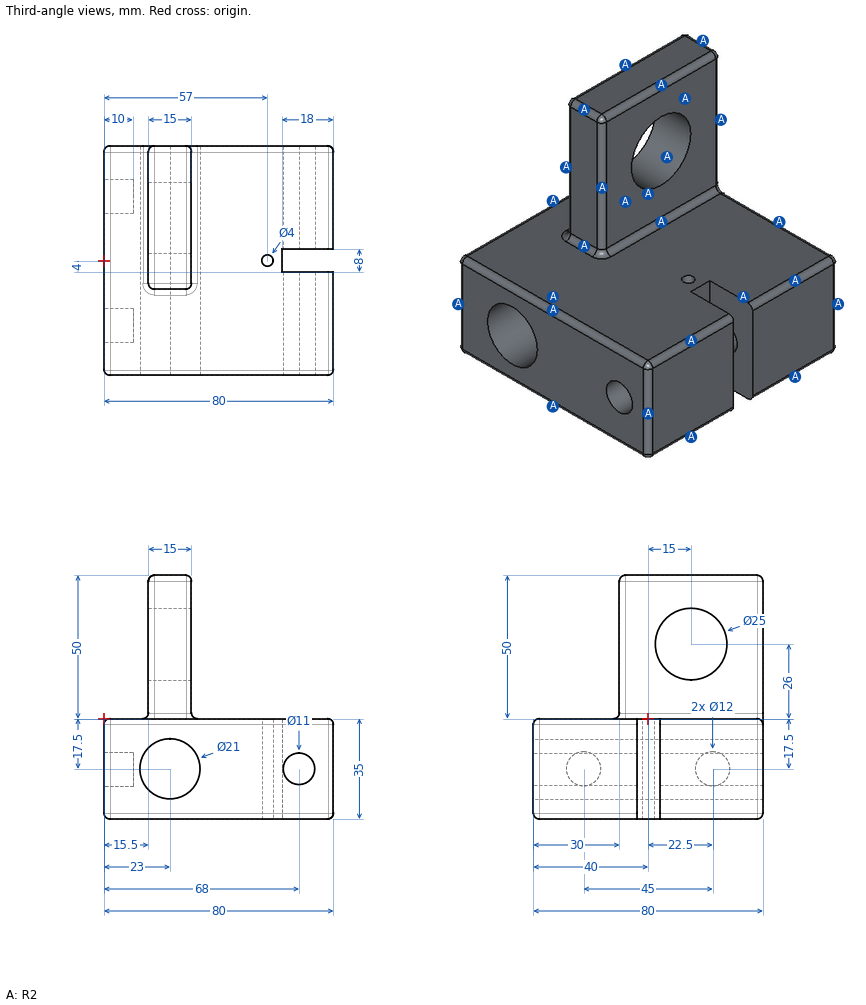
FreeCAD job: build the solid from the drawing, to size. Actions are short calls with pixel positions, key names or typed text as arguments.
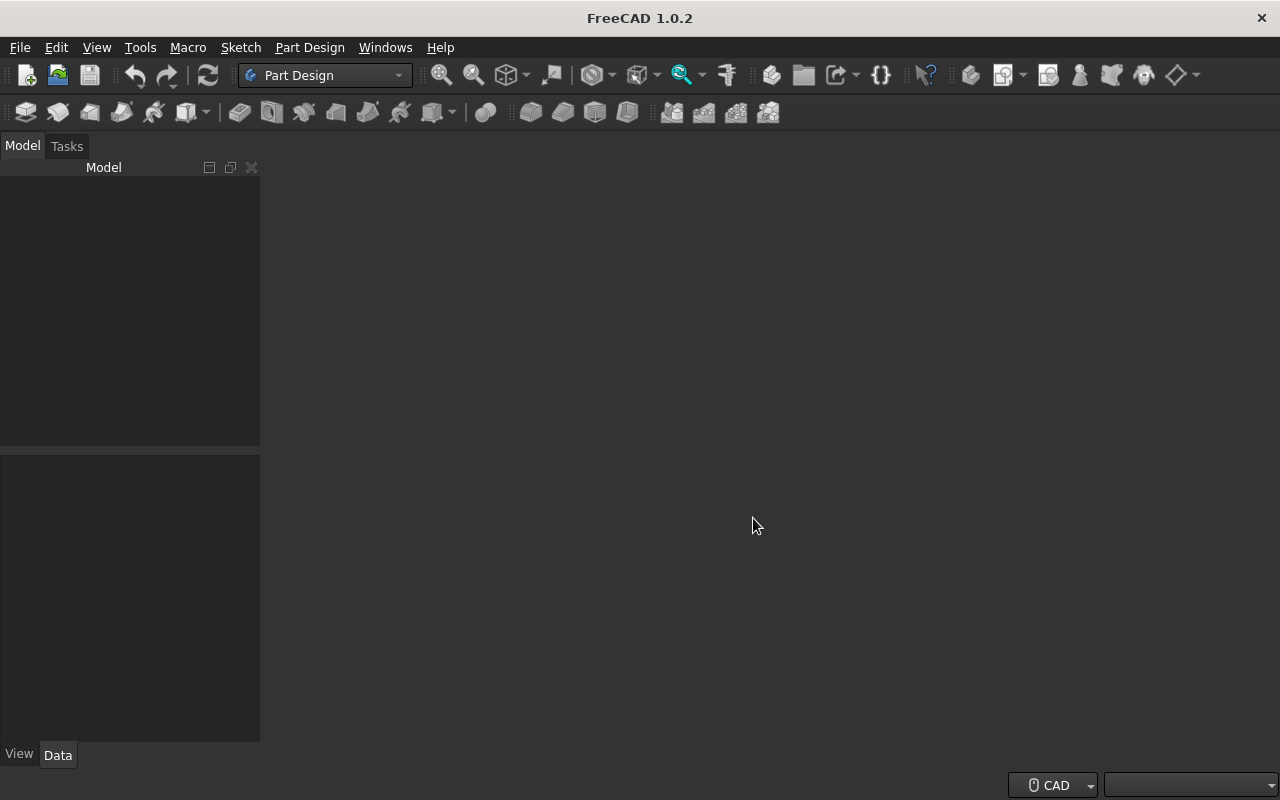
click(26, 76)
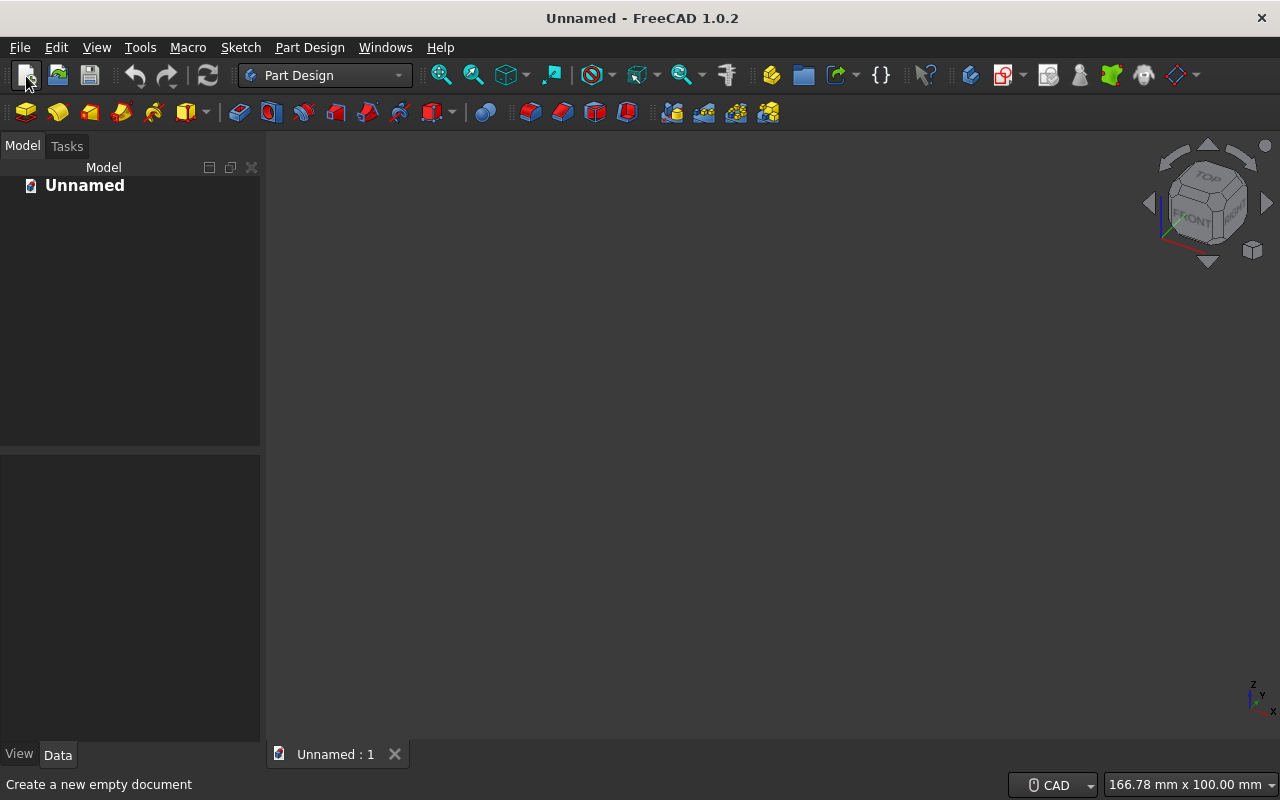
click(1004, 76)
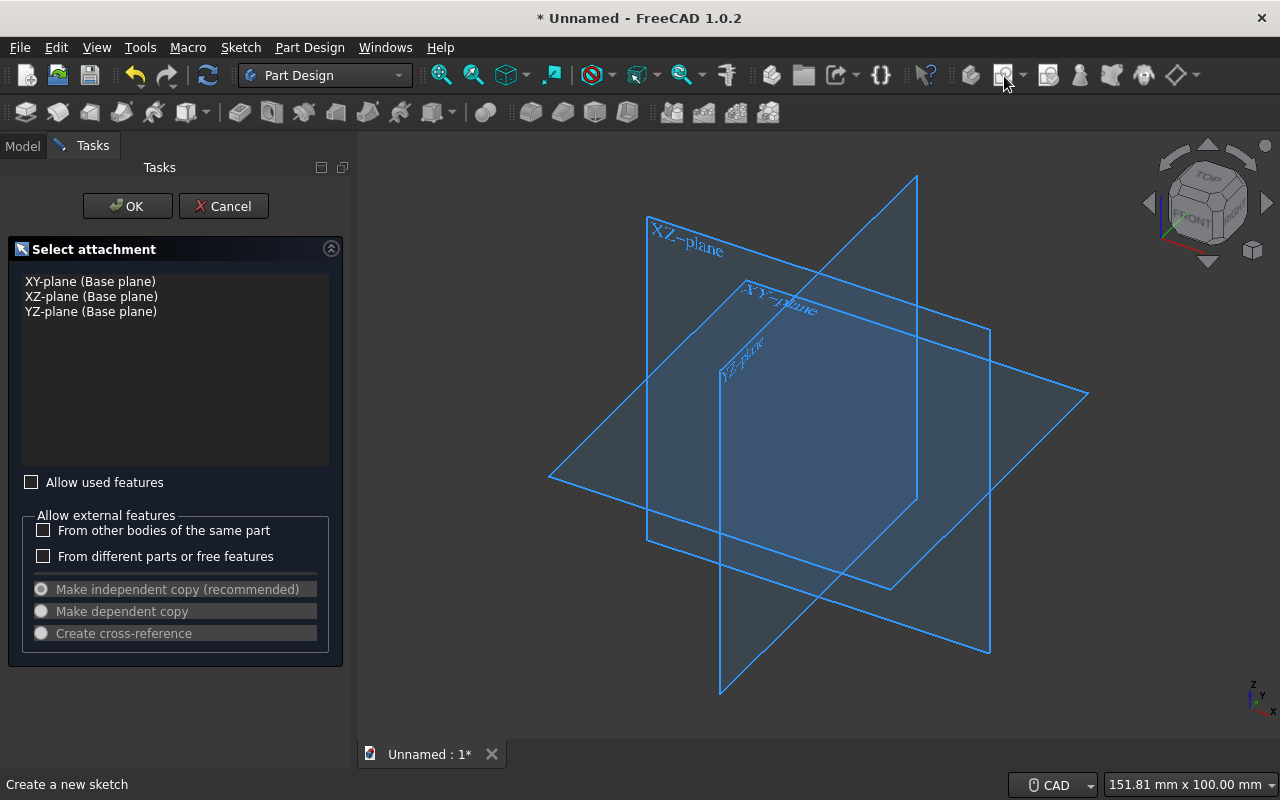
click(82, 296)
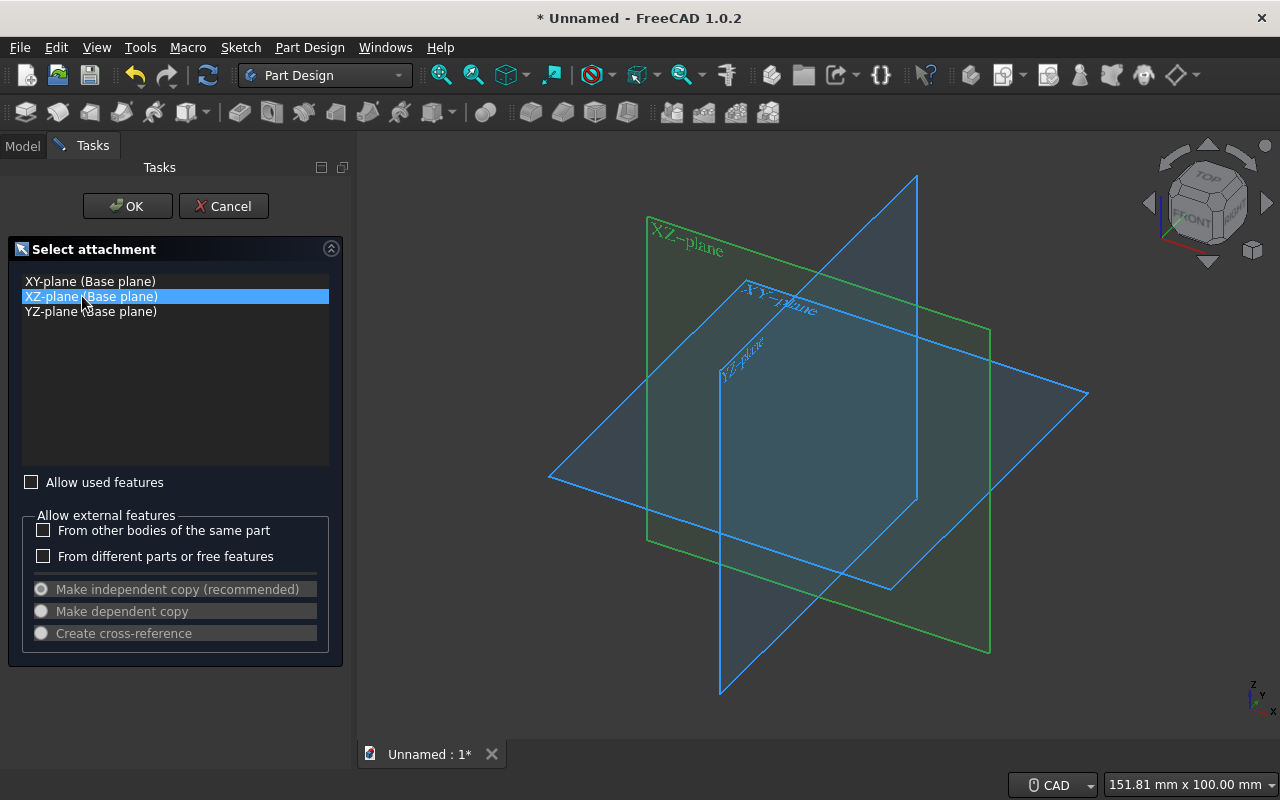
click(128, 206)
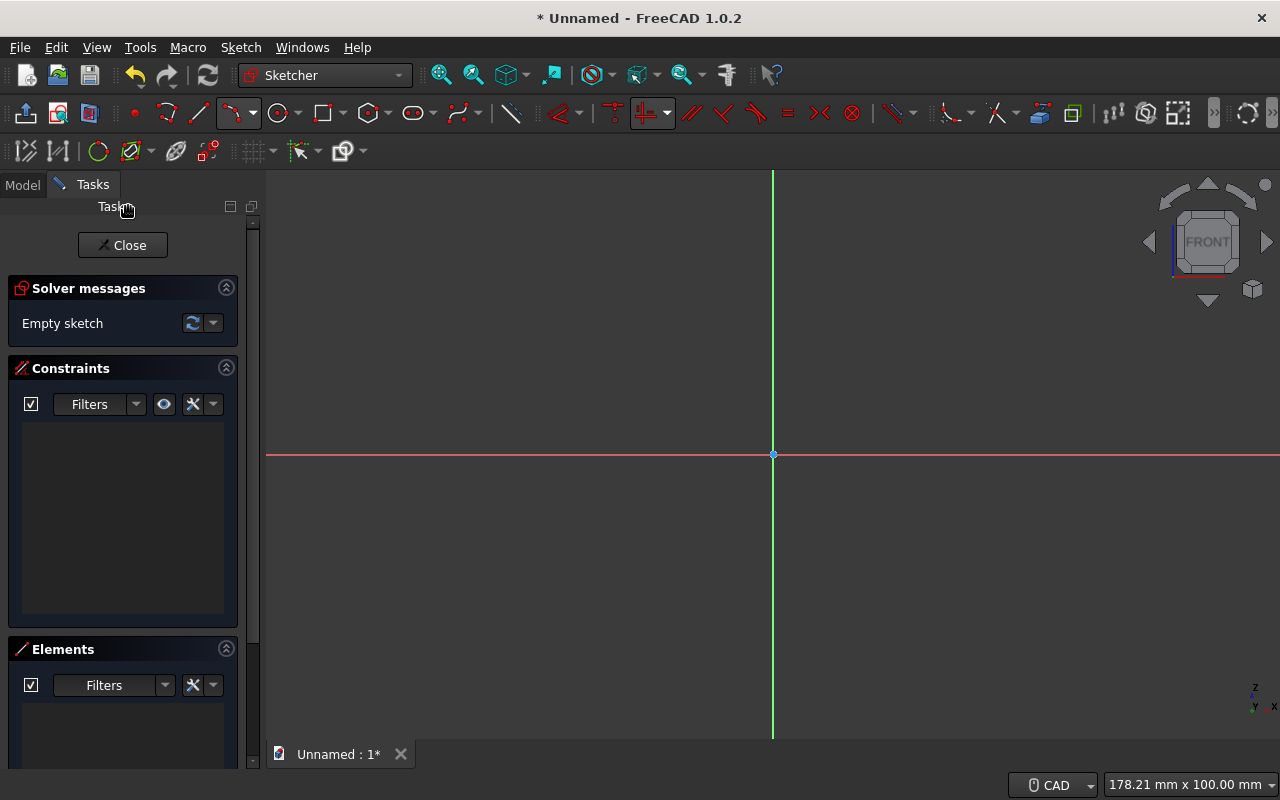
scroll(294, 647, down, 1)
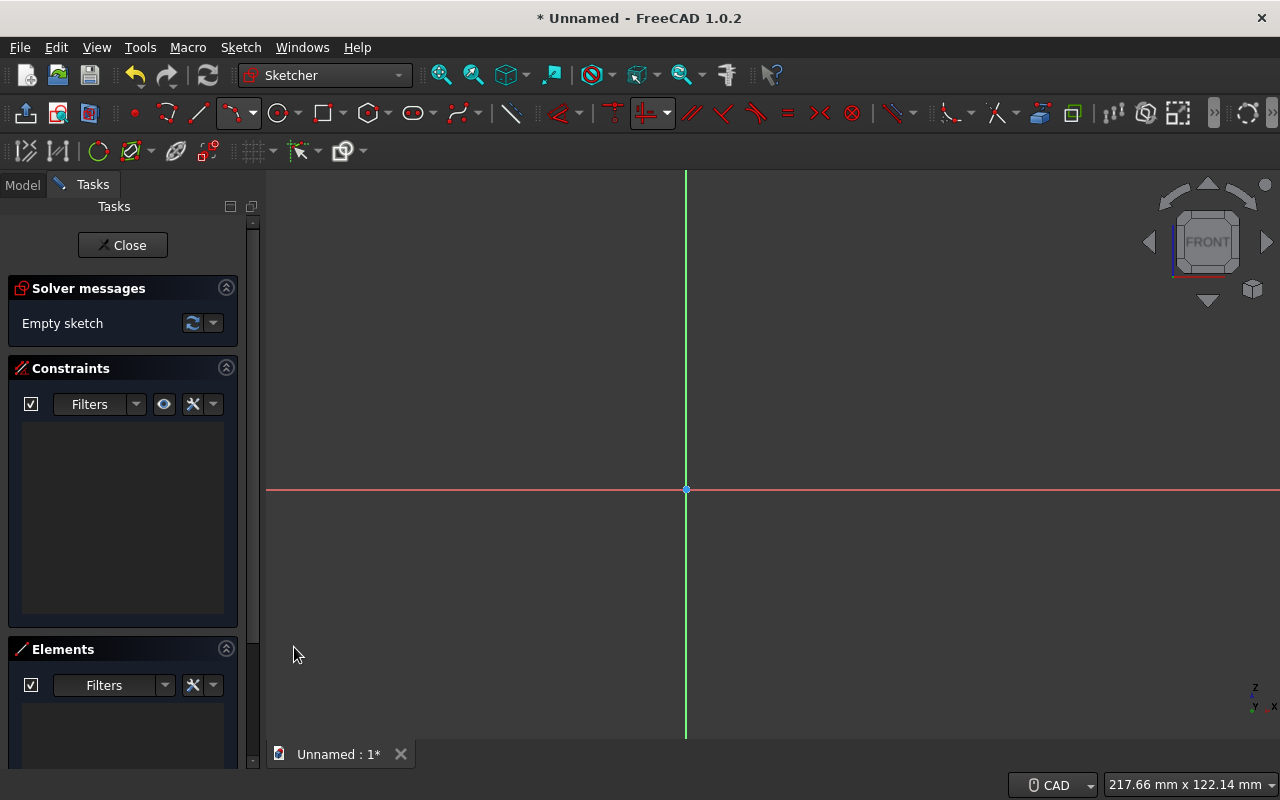
click(168, 114)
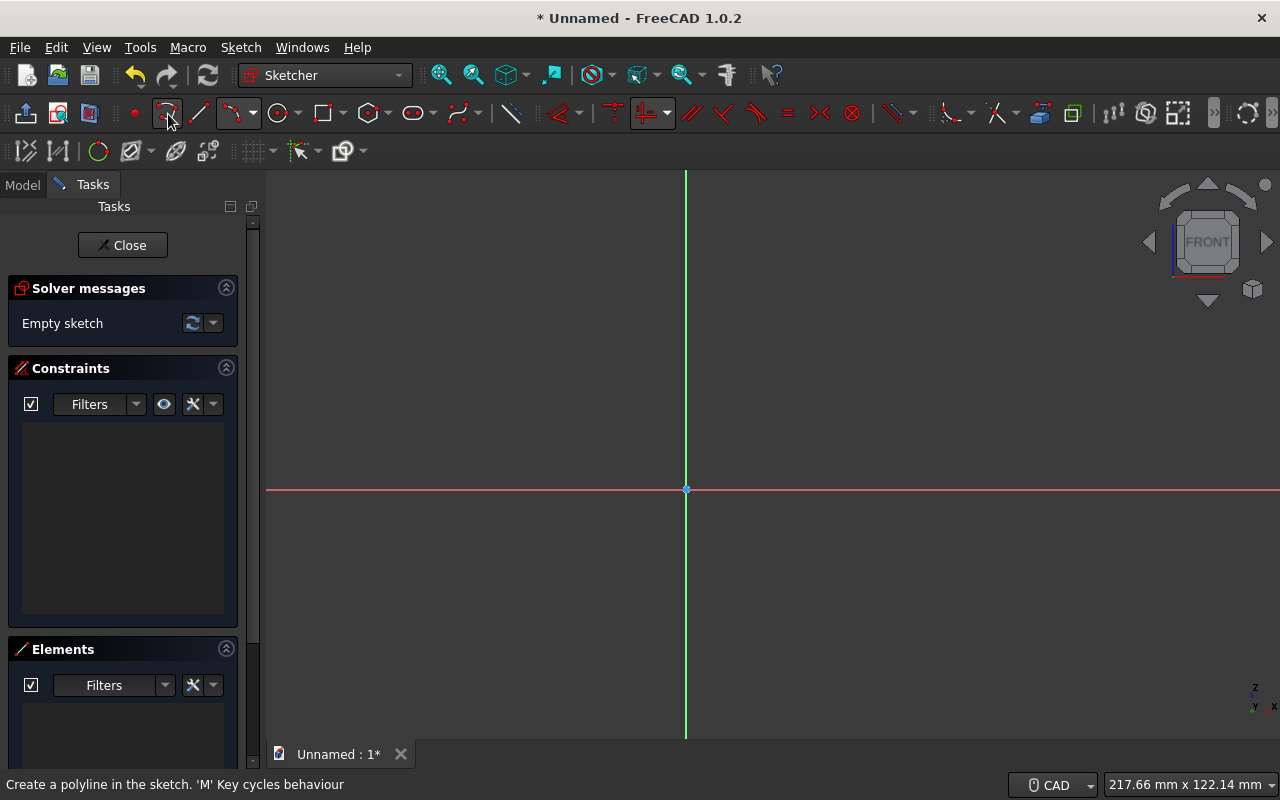
click(686, 490)
click(758, 481)
click(758, 257)
click(828, 257)
click(828, 490)
click(1059, 481)
click(1059, 653)
click(695, 653)
click(686, 490)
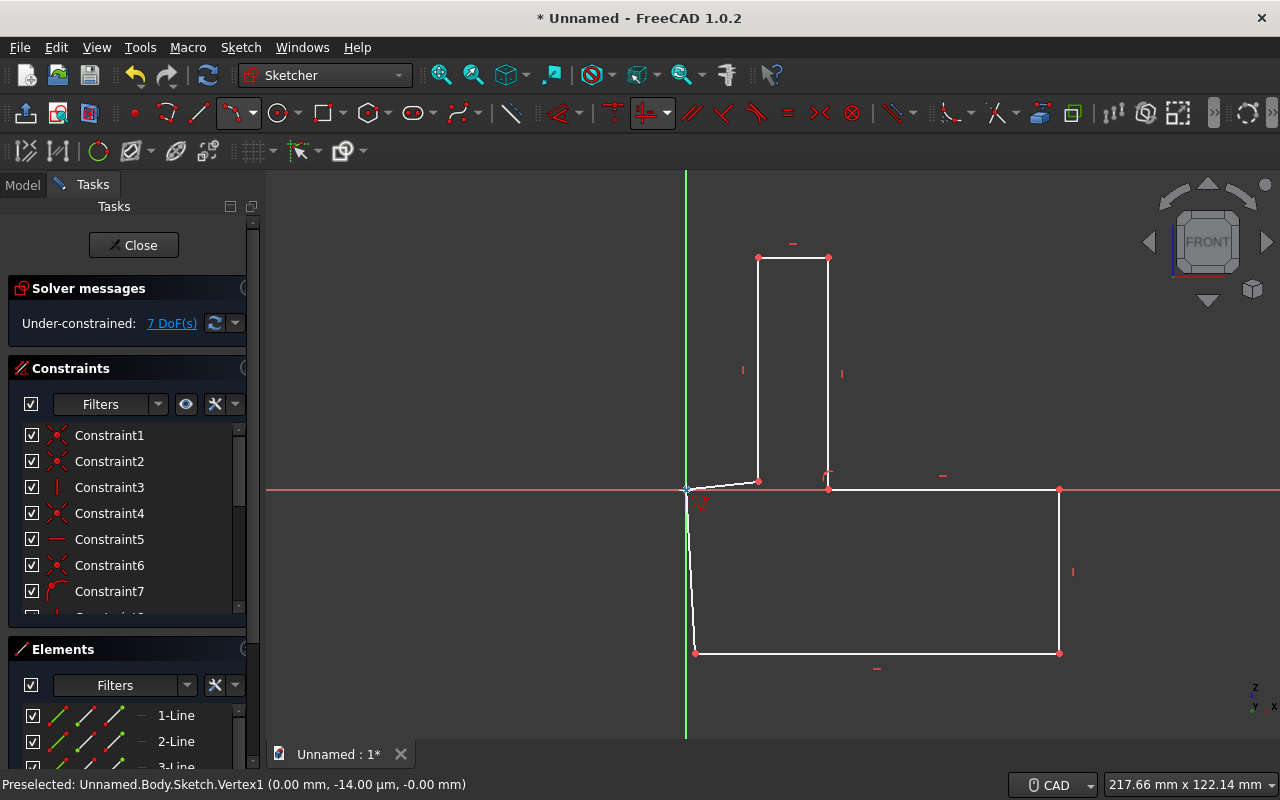
click(278, 114)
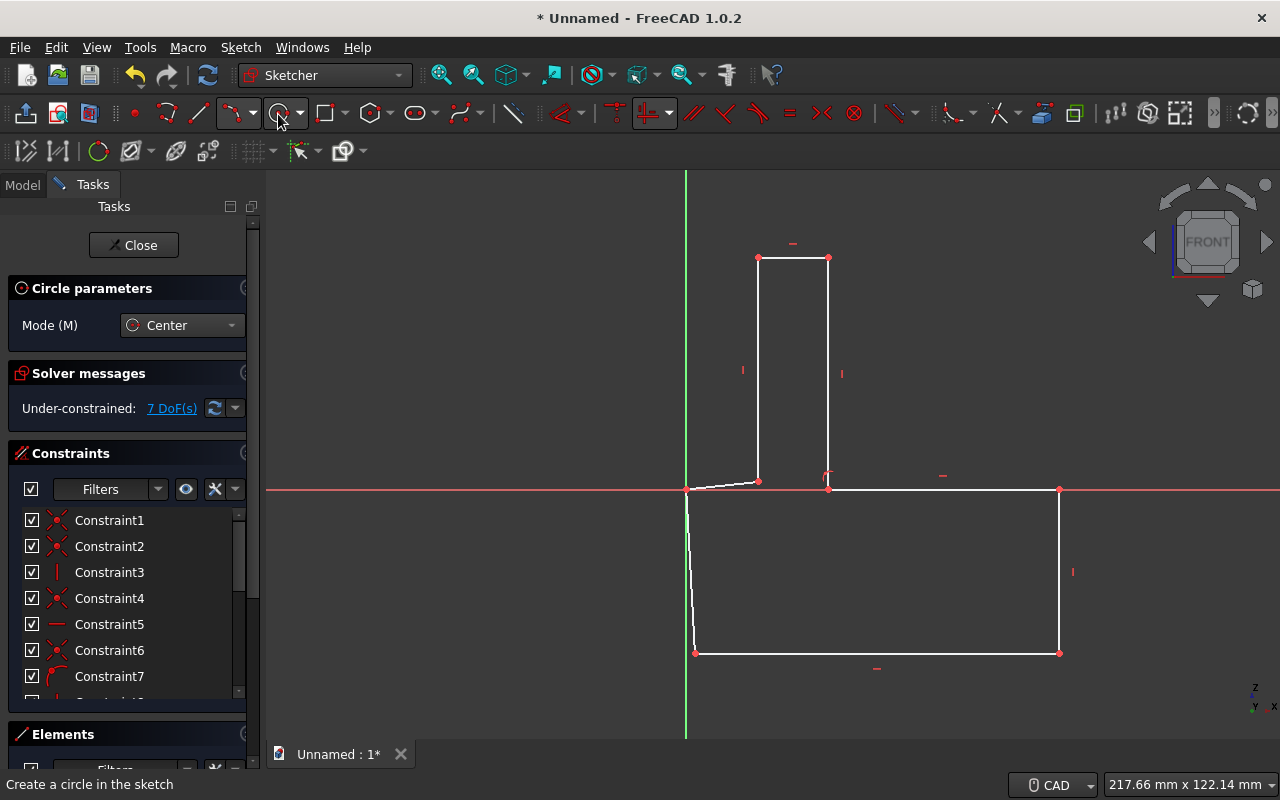
click(793, 571)
click(828, 536)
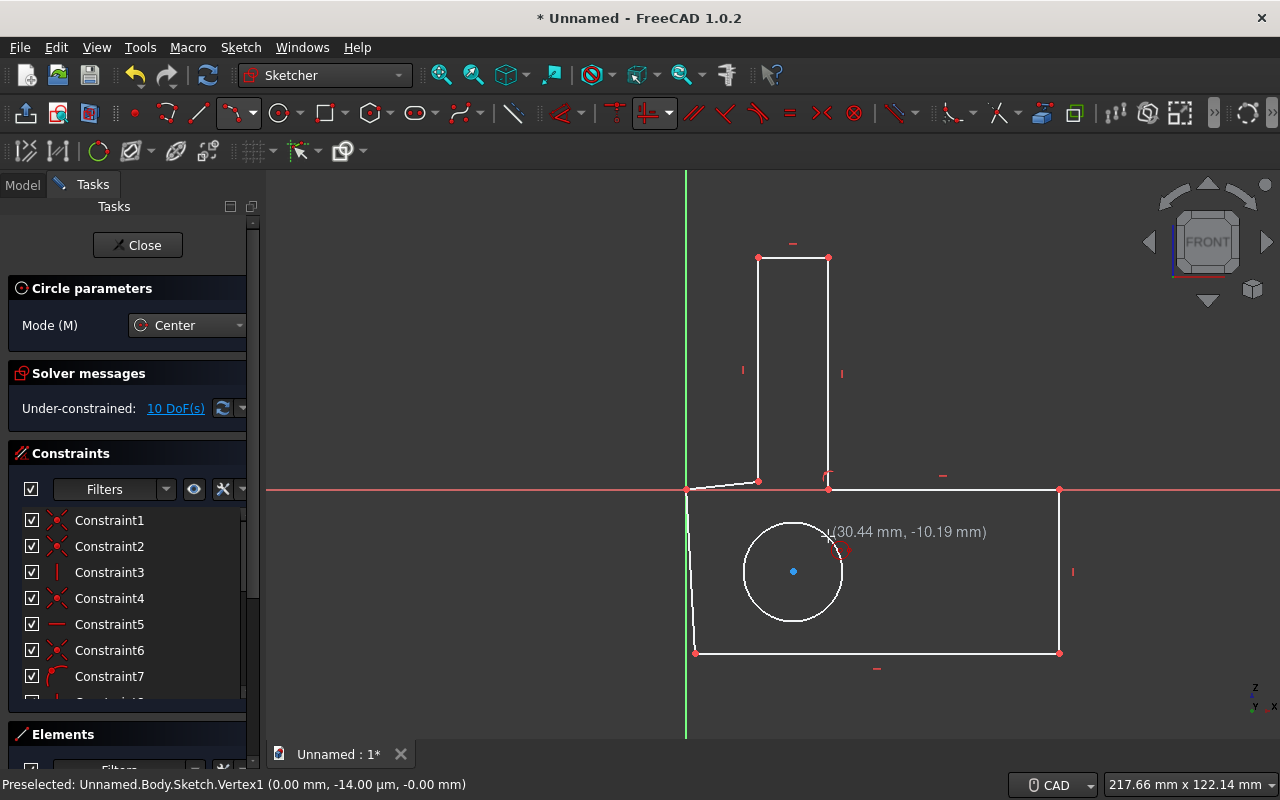
click(1003, 571)
click(1021, 553)
key(Escape)